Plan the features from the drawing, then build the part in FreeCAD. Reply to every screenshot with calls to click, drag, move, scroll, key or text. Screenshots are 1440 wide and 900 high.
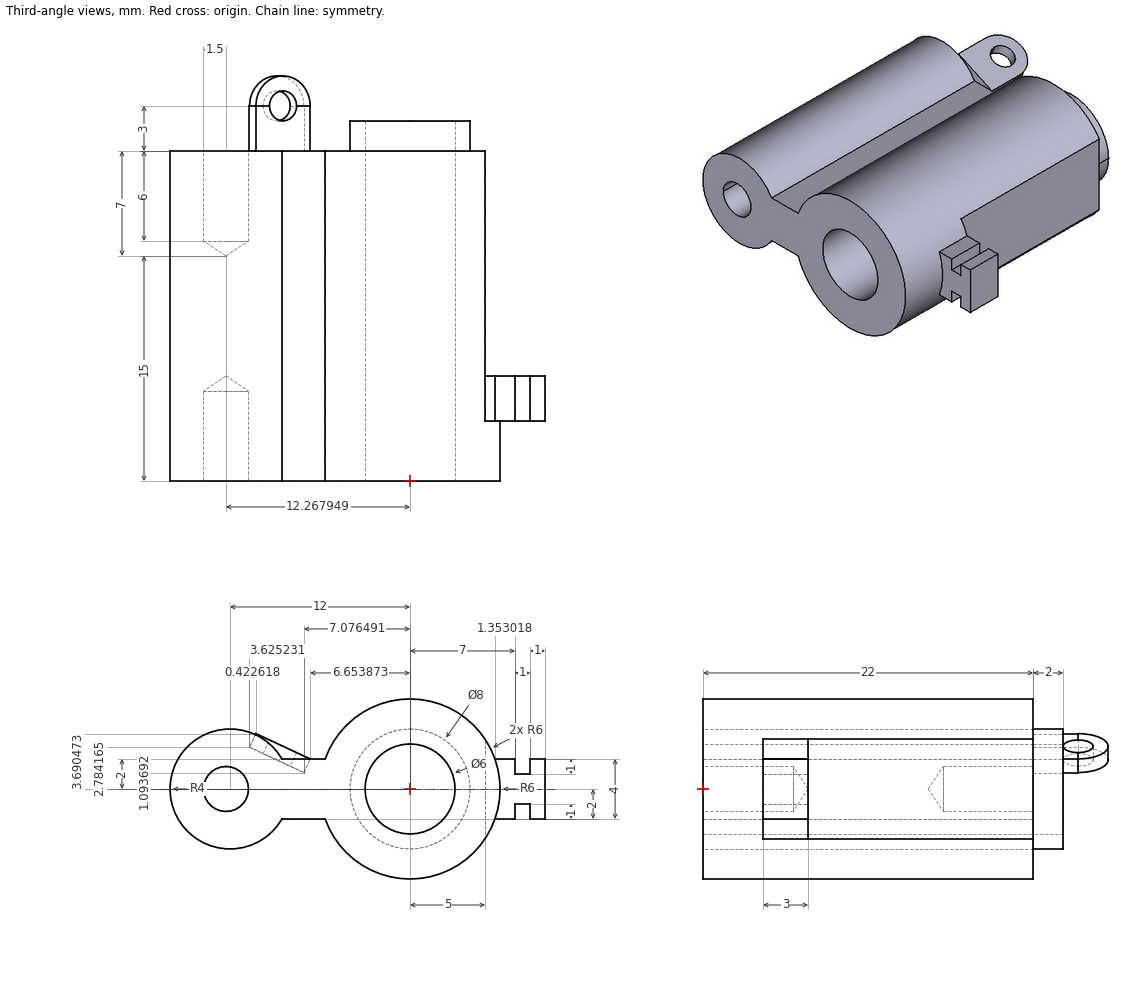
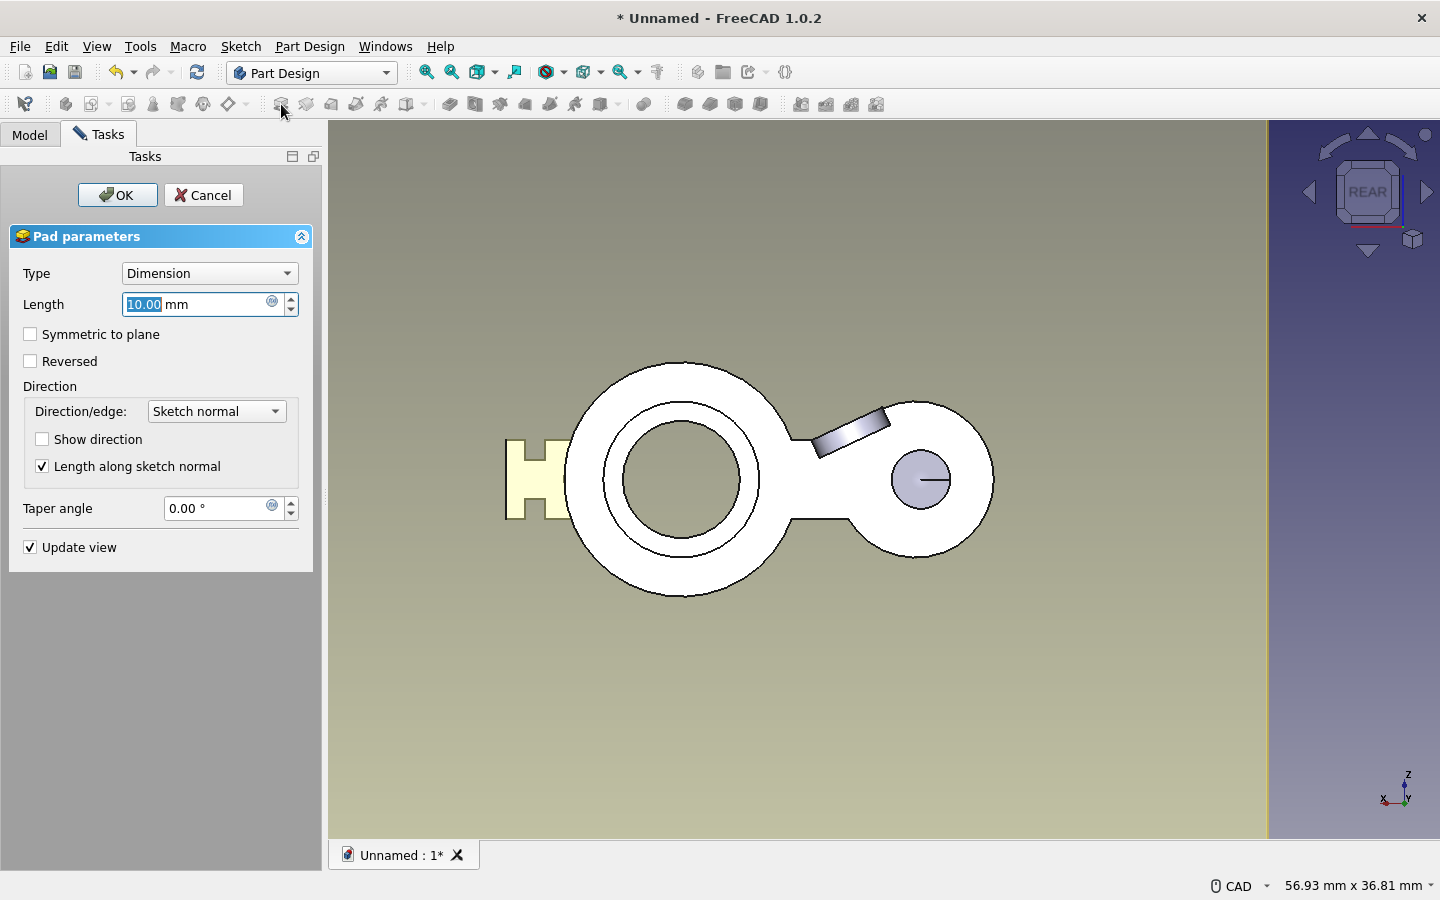
text(3)
key(Tab)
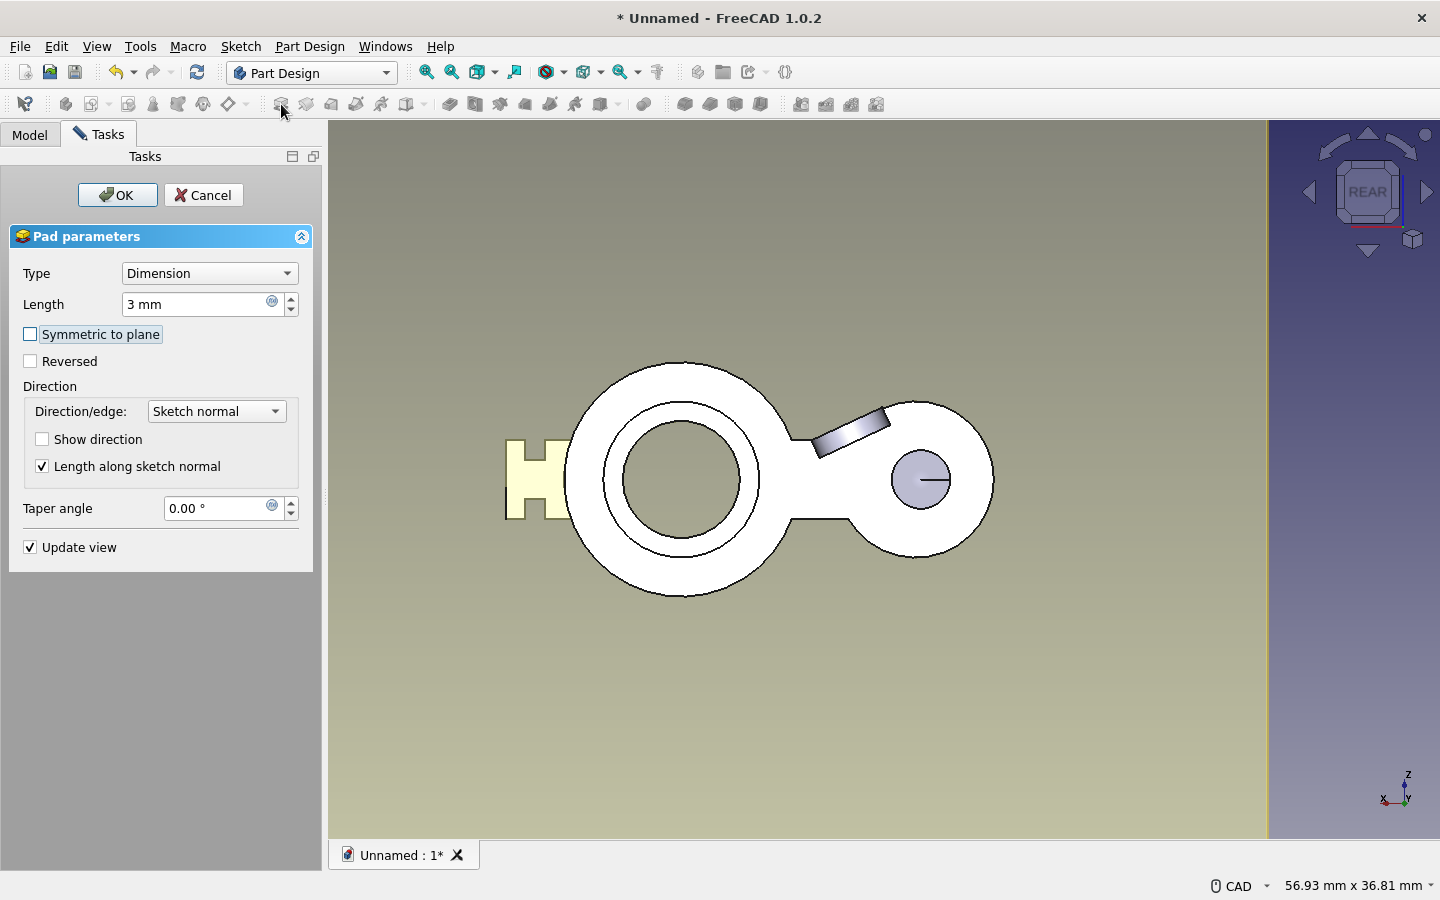
click(31, 361)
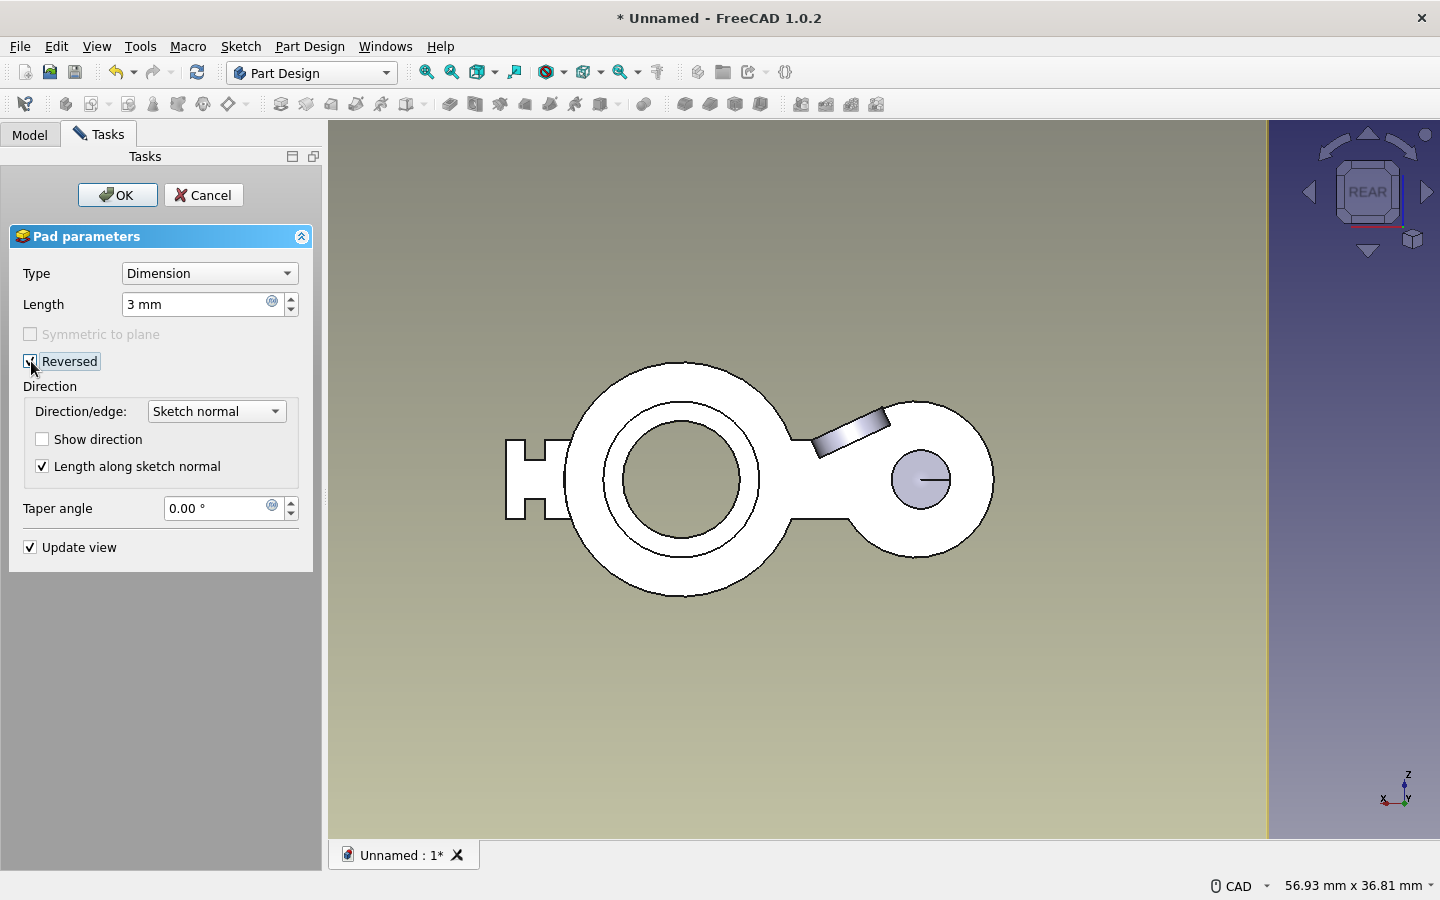
click(118, 195)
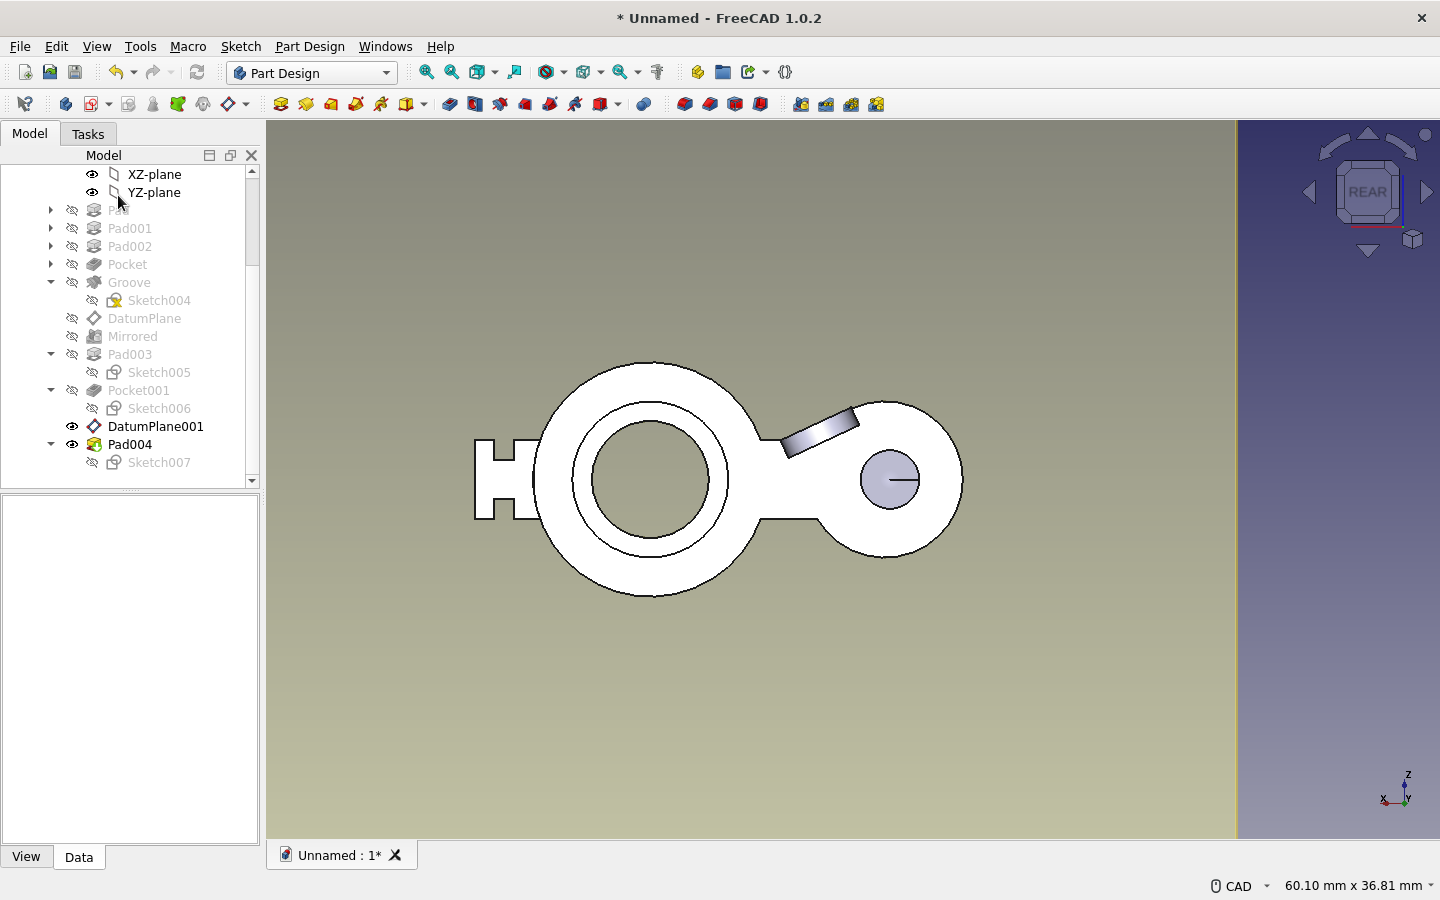
click(117, 426)
key(space)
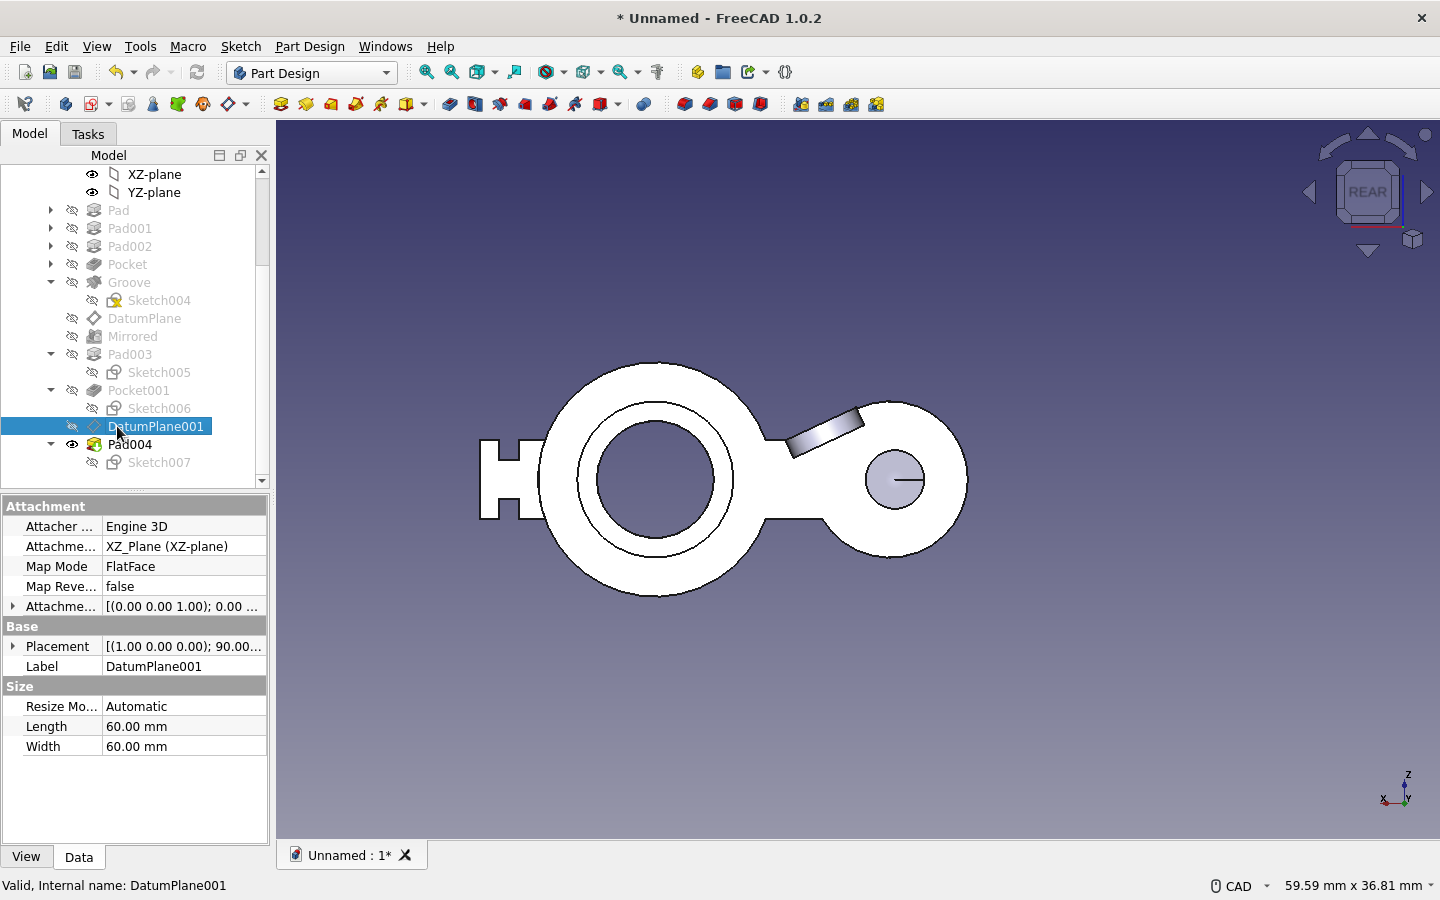
click(427, 72)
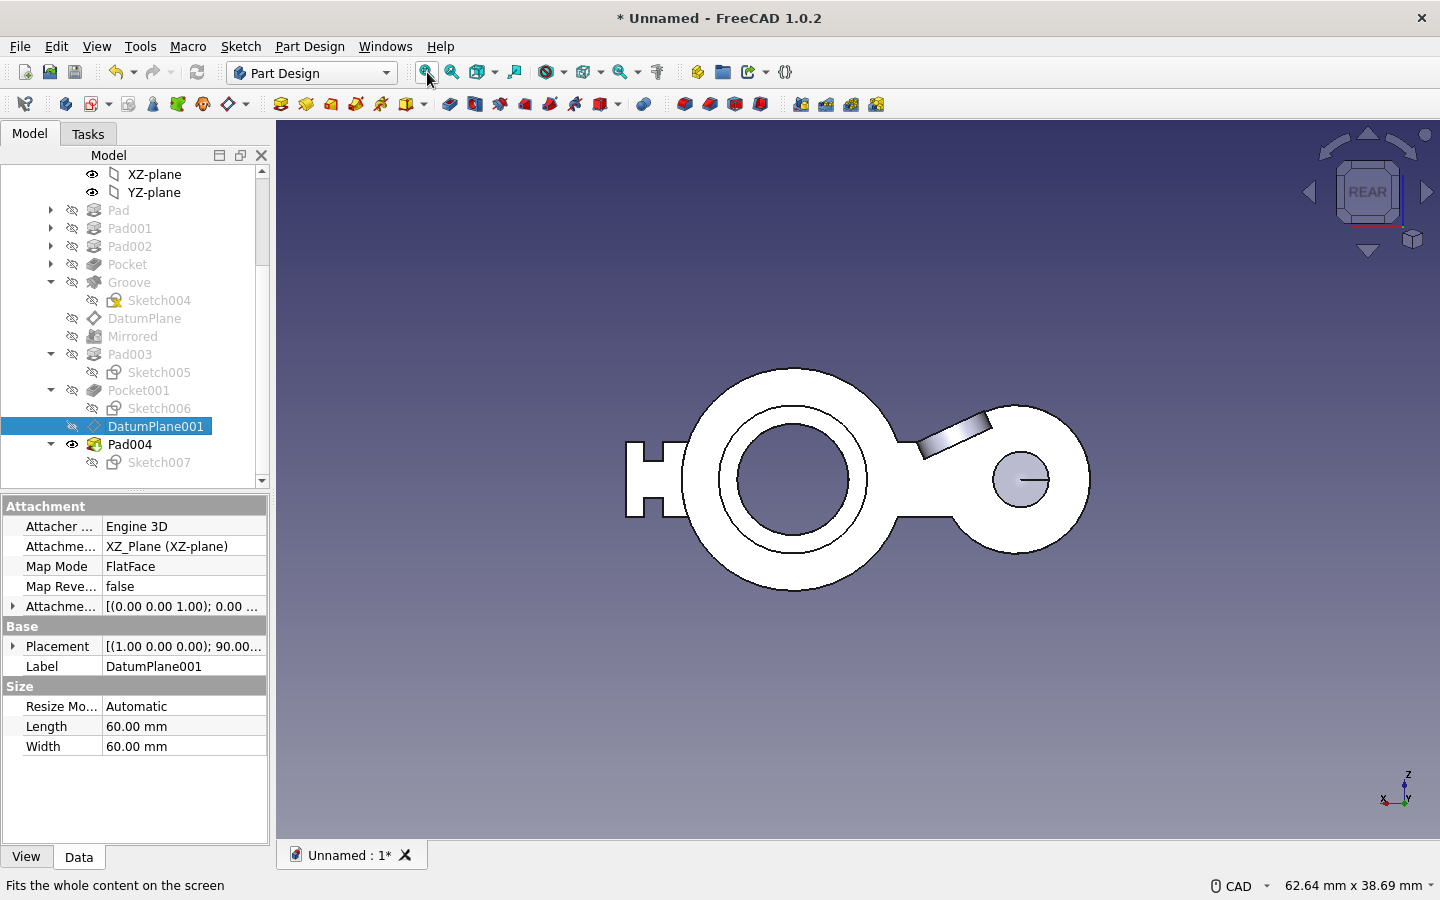
click(648, 478)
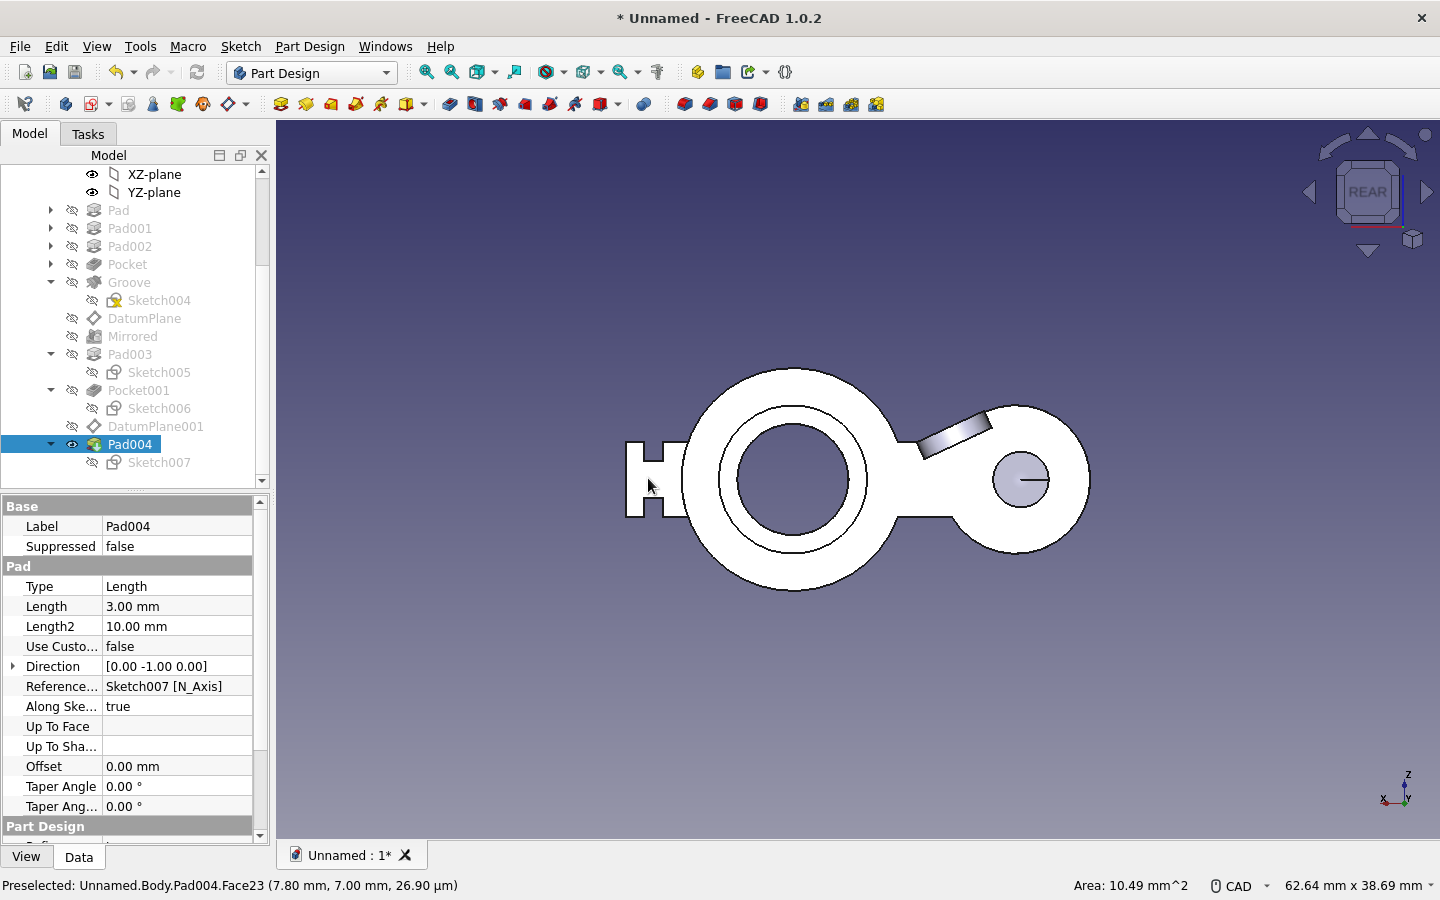
click(90, 104)